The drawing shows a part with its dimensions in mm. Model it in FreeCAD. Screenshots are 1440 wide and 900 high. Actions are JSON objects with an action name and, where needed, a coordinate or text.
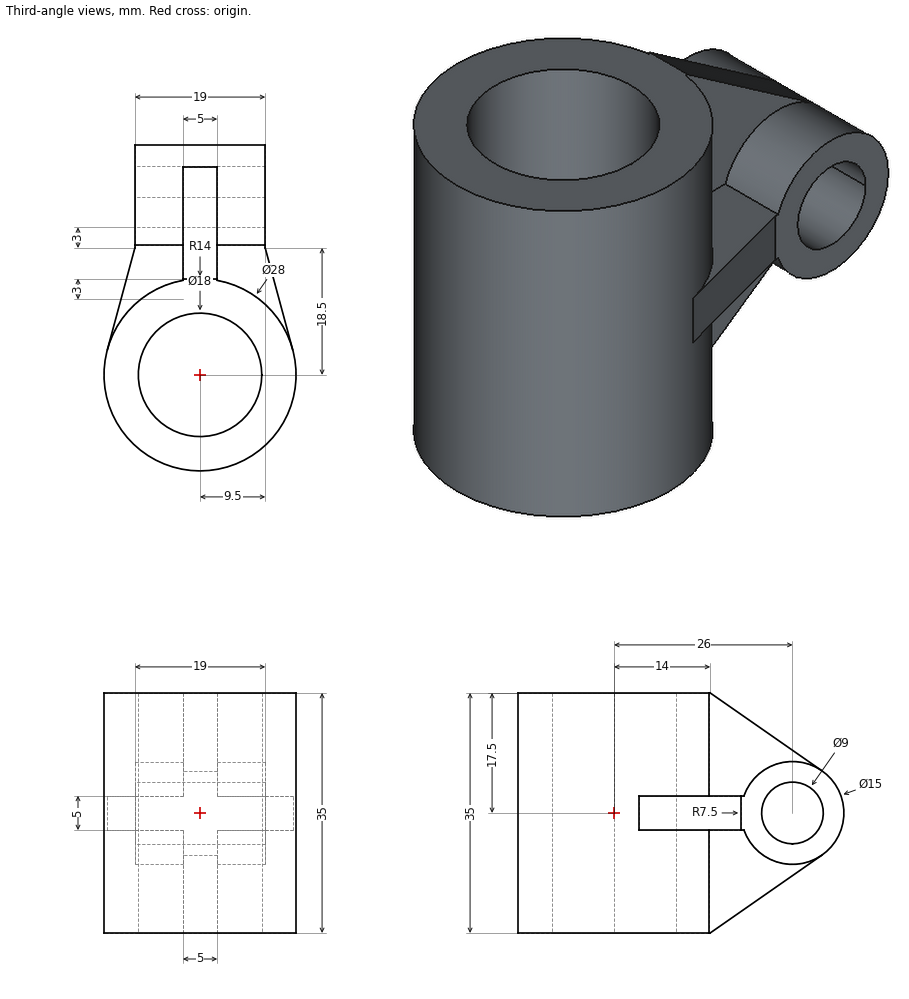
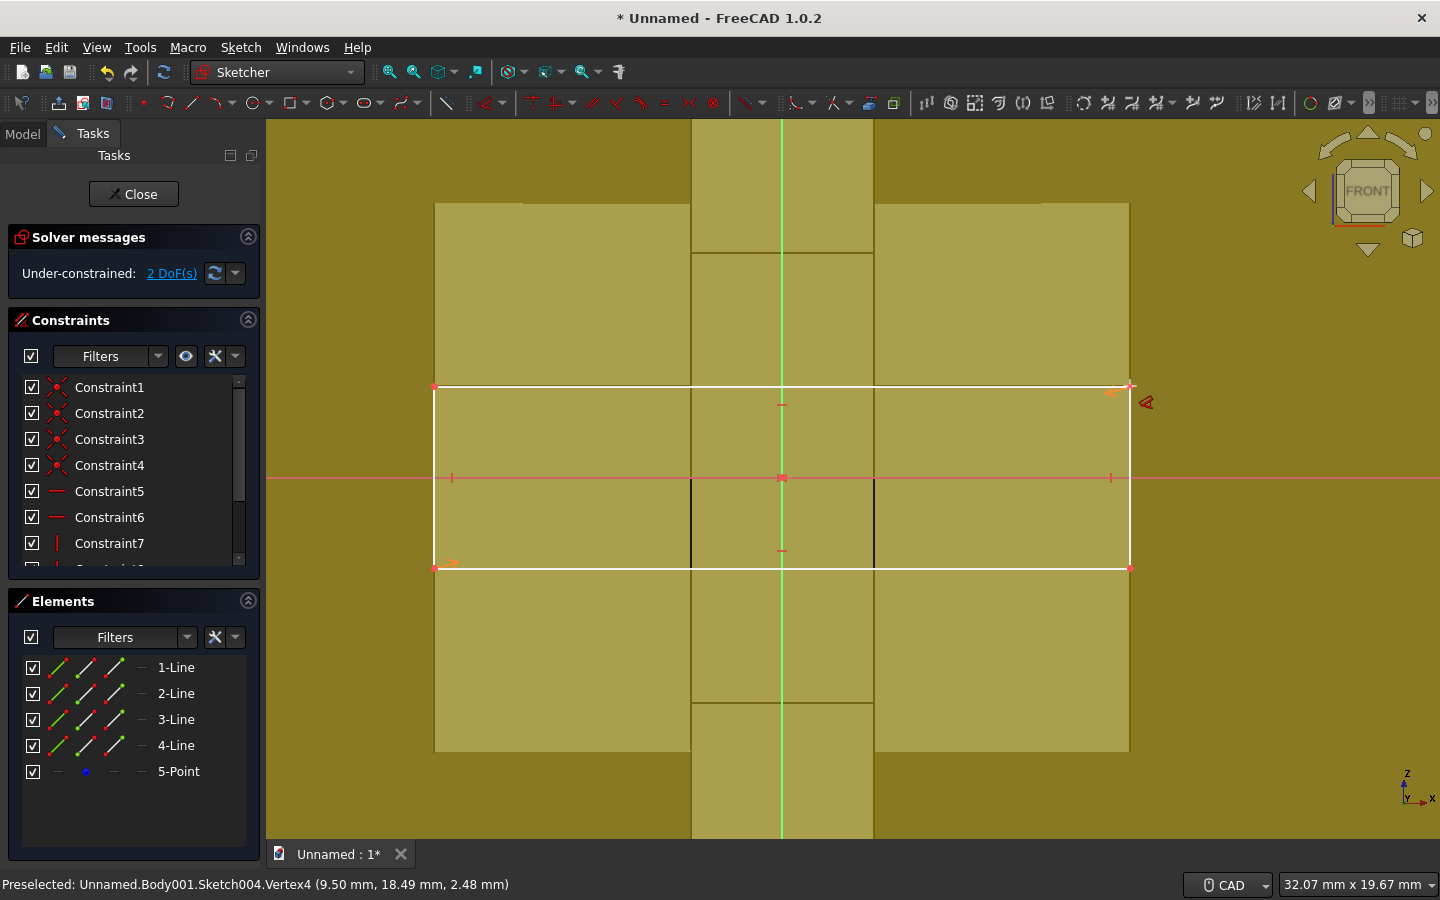
{"action": "left_click", "coordinate": [1130, 514]}
{"action": "left_click", "coordinate": [1164, 436]}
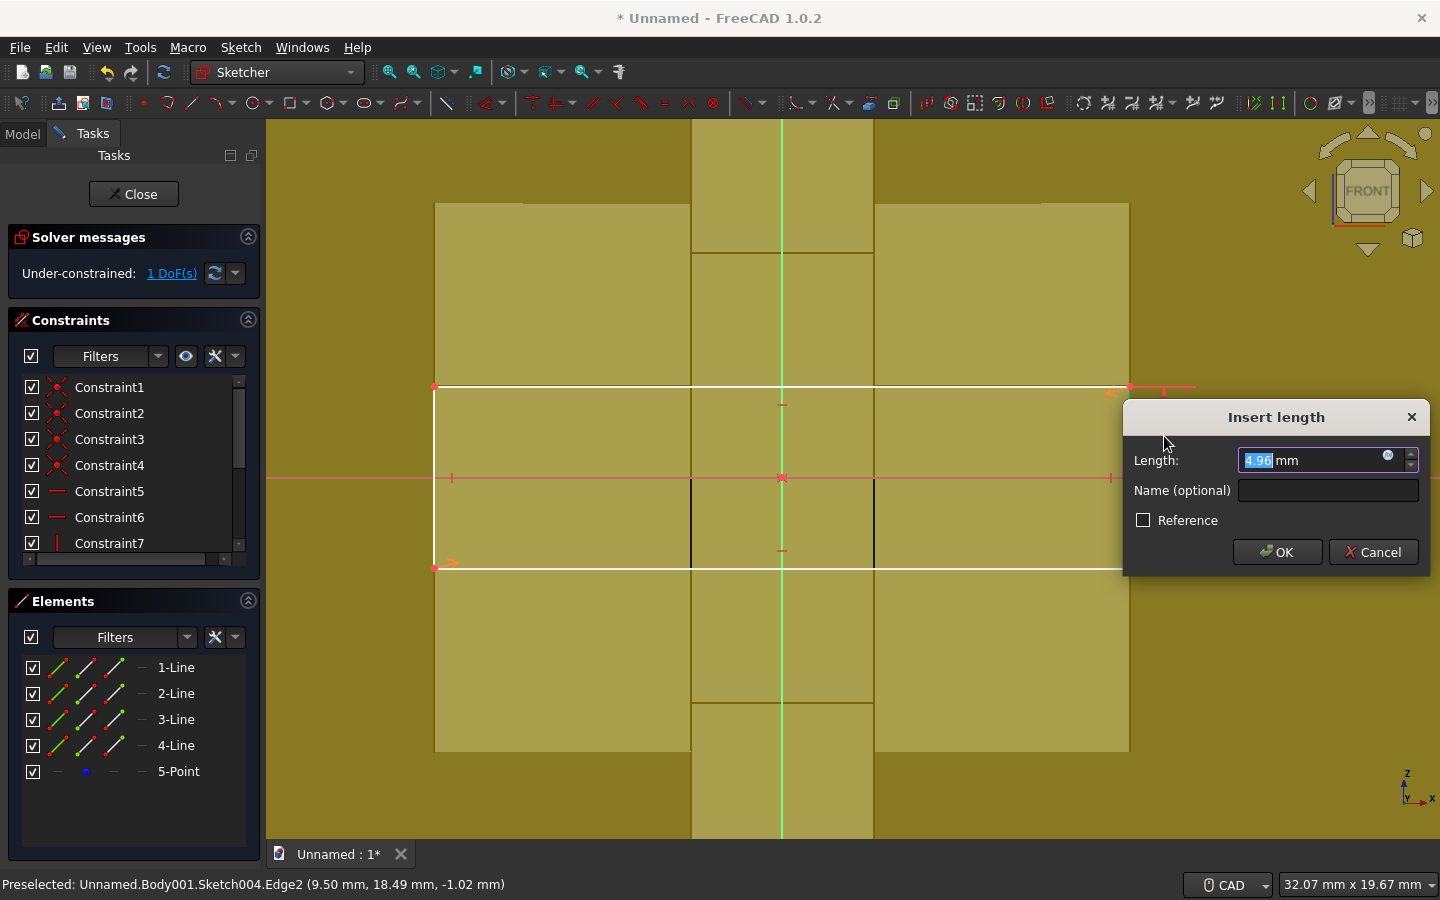
{"action": "type", "text": "5"}
{"action": "key", "text": "Return"}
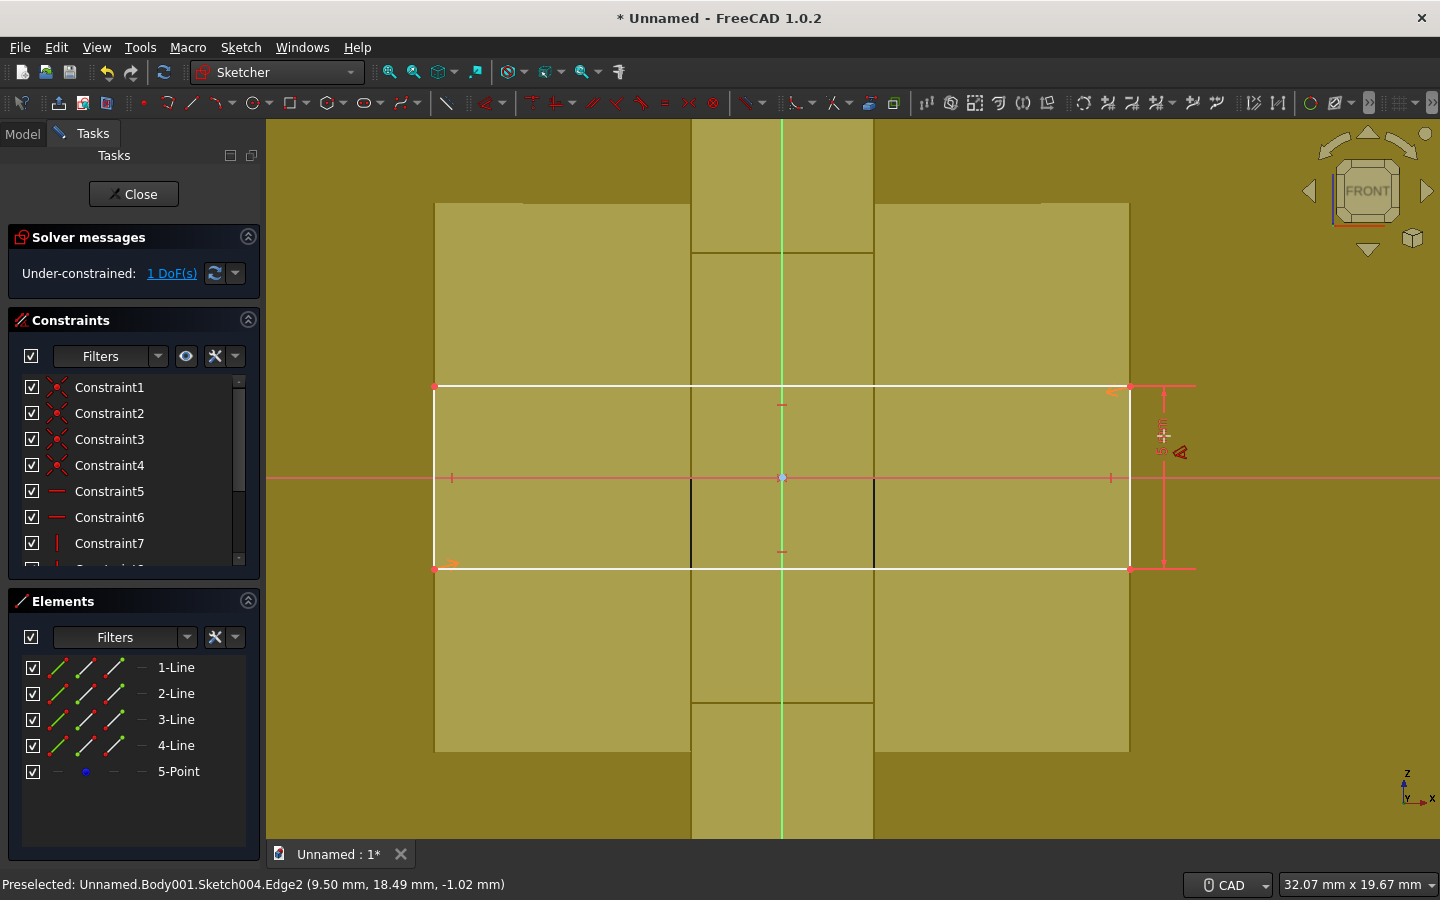
{"action": "left_click", "coordinate": [643, 569]}
{"action": "left_click", "coordinate": [622, 603]}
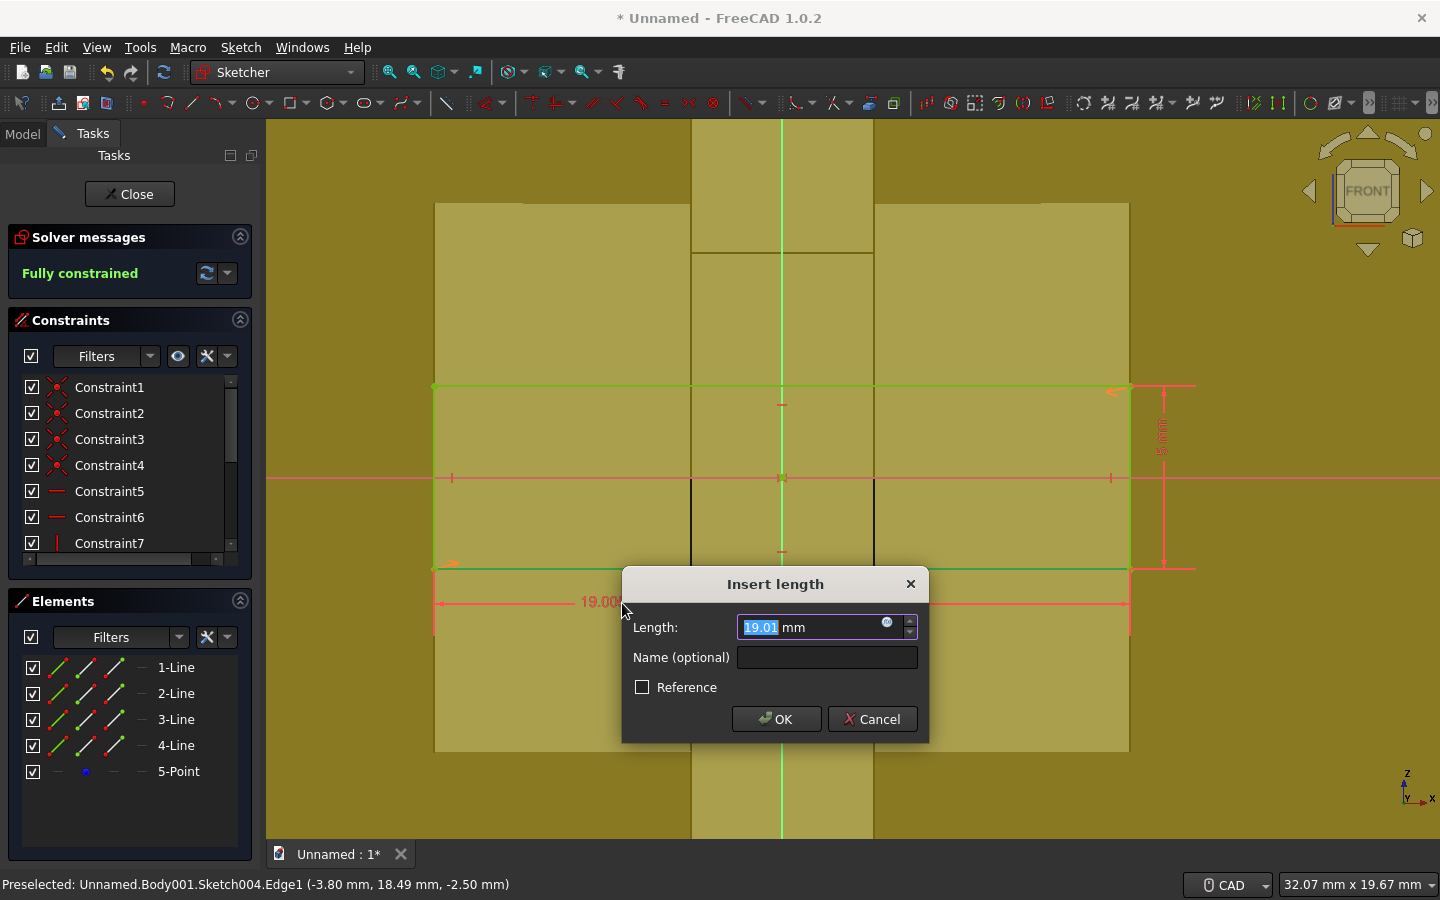
{"action": "type", "text": "19"}
{"action": "key", "text": "Return"}
{"action": "key", "text": "Escape"}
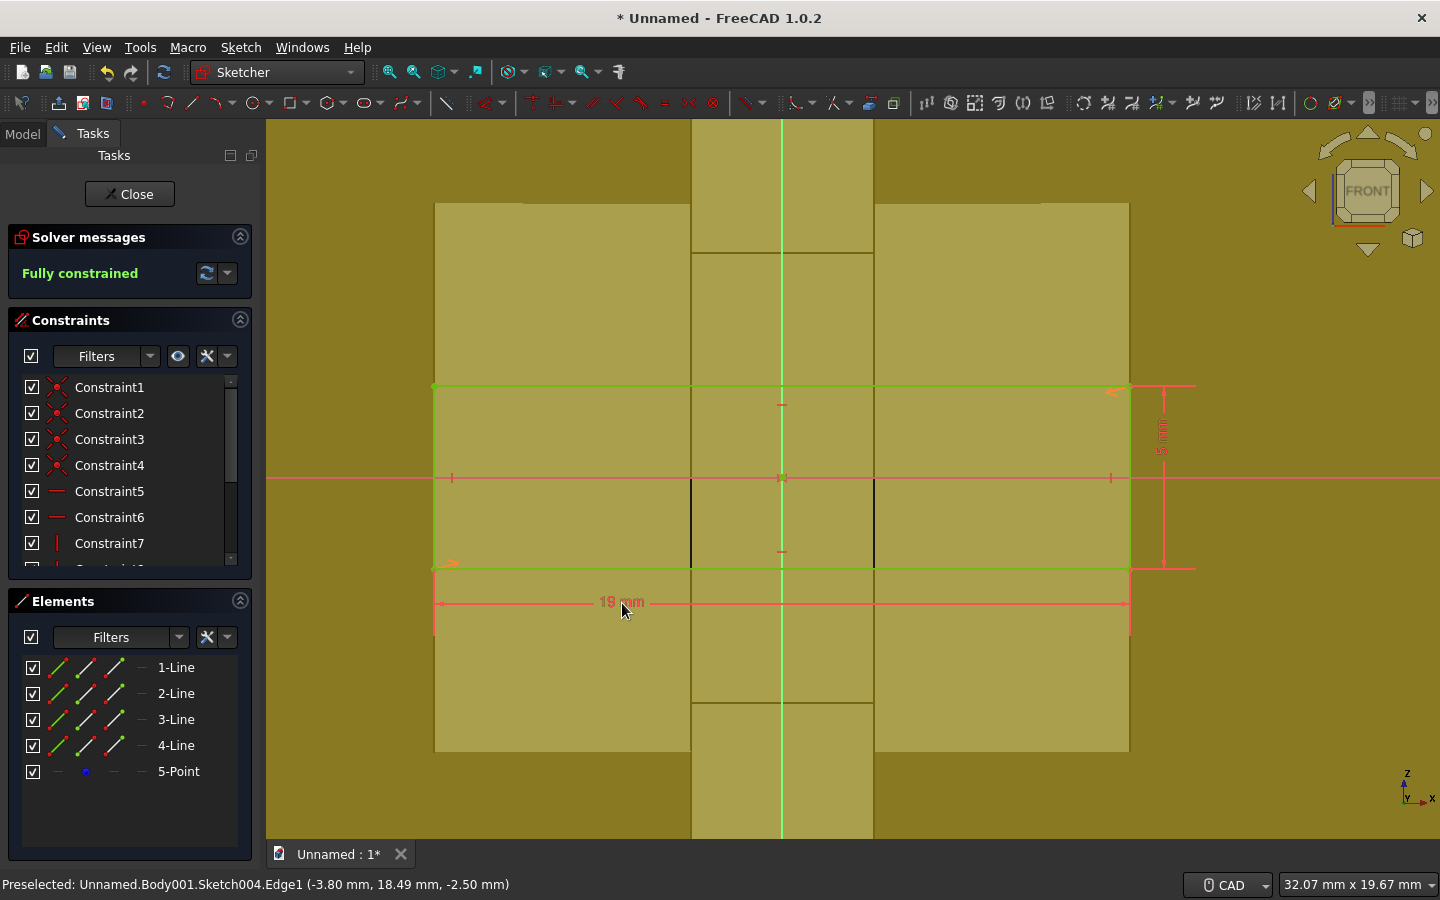
{"action": "left_click", "coordinate": [130, 194]}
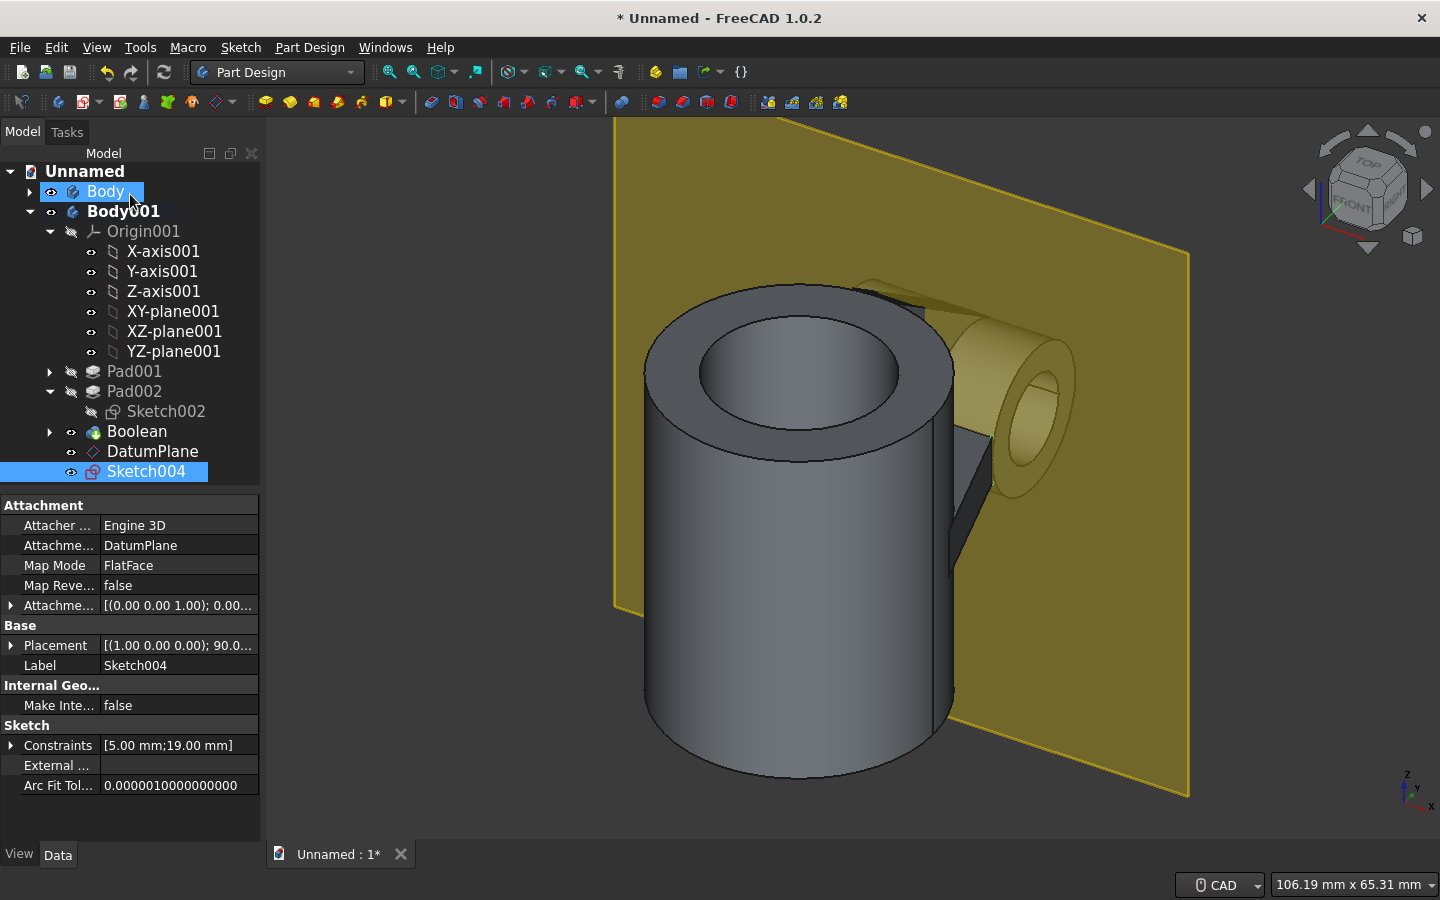
{"action": "left_click", "coordinate": [266, 102]}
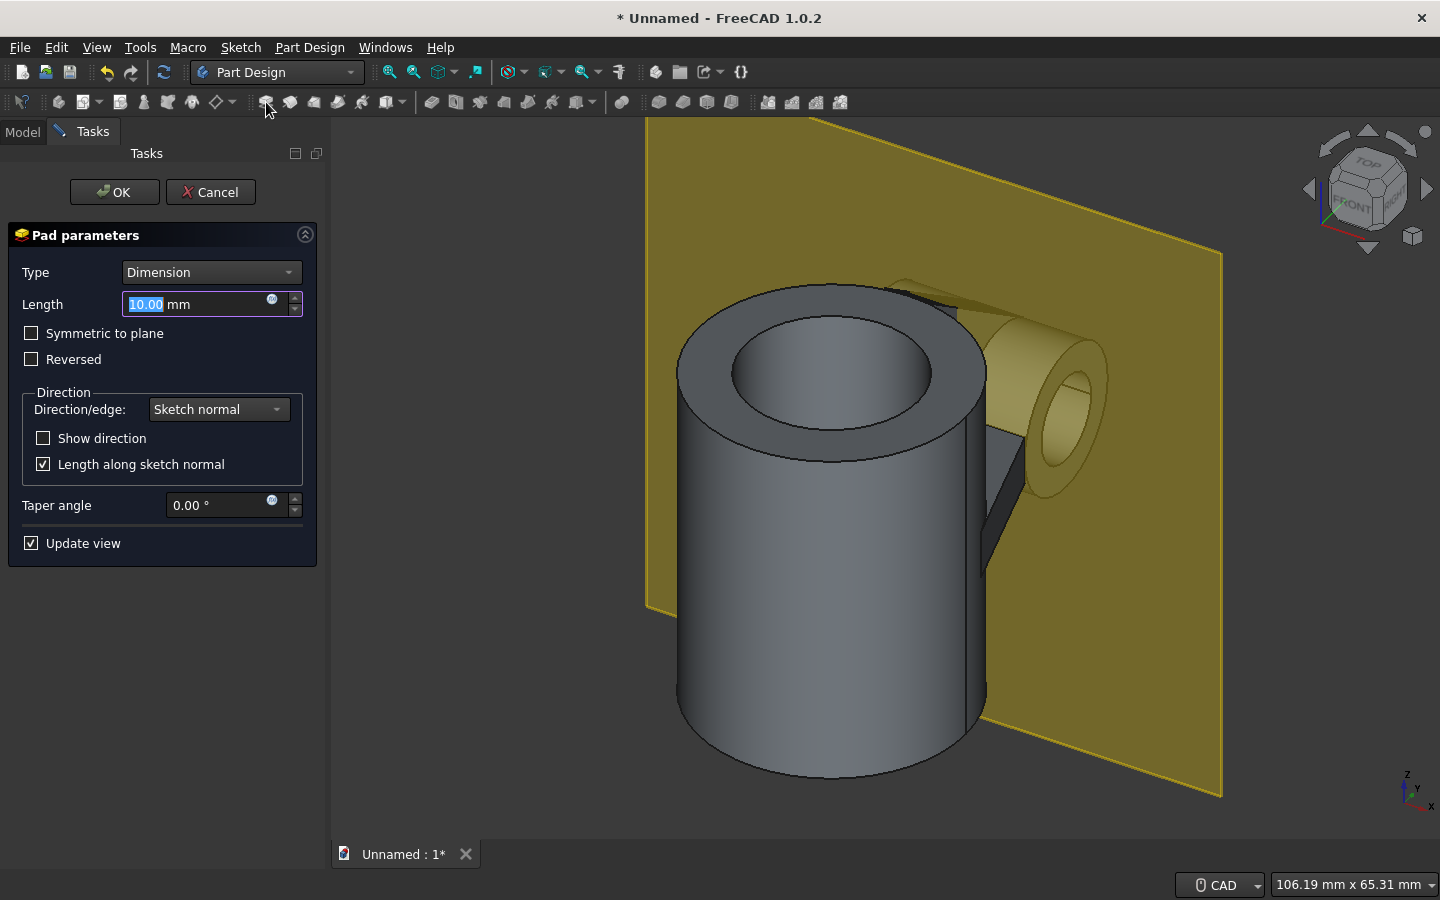
{"action": "type", "text": "3"}
{"action": "key", "text": "Tab"}